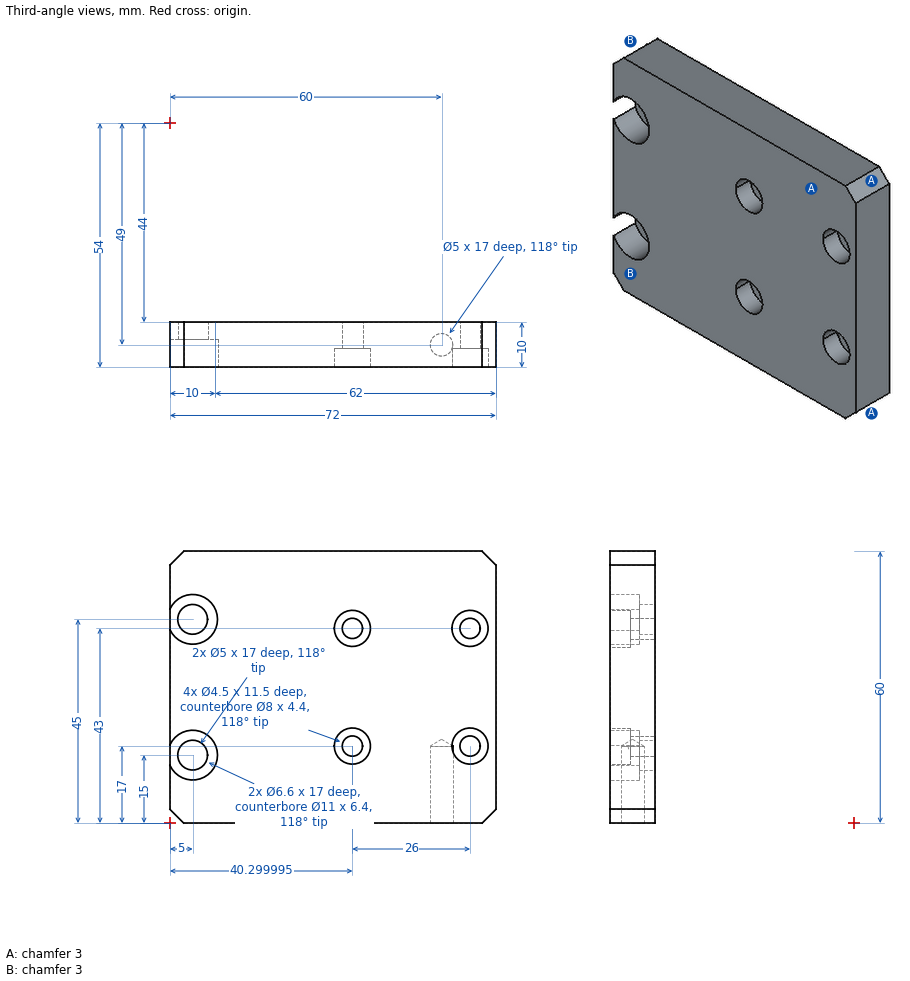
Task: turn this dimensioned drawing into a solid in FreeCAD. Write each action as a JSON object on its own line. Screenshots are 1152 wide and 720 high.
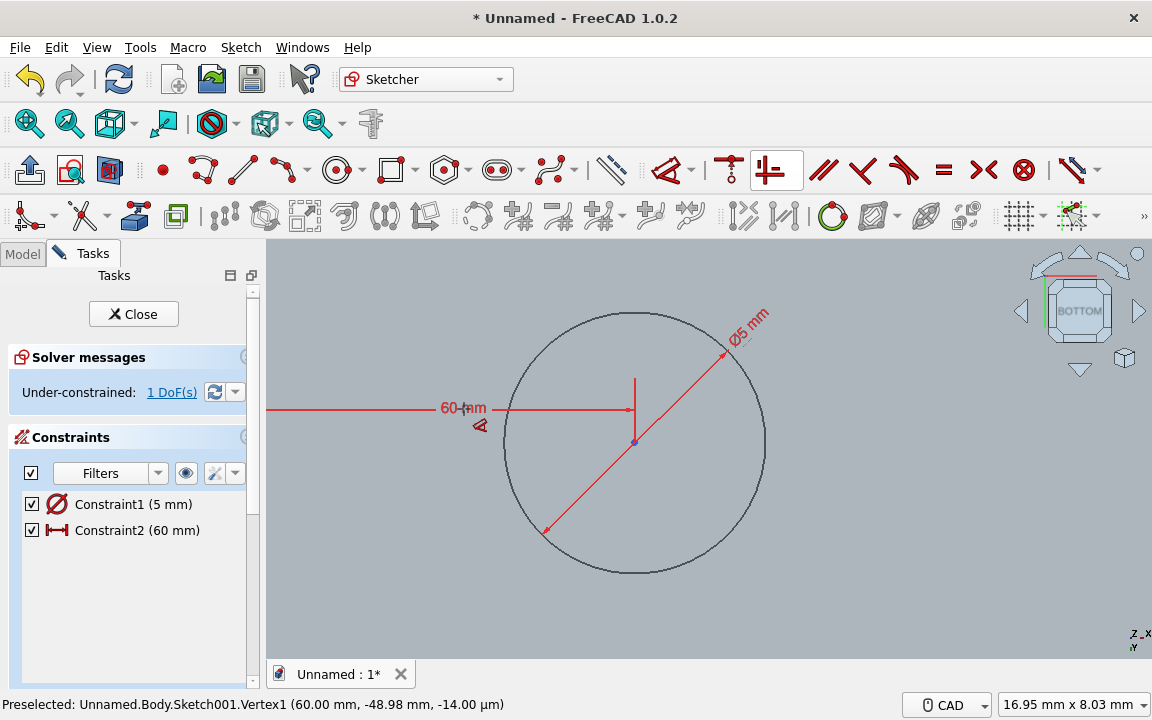
{"action": "left_click", "coordinate": [635, 443]}
{"action": "left_click", "coordinate": [669, 537]}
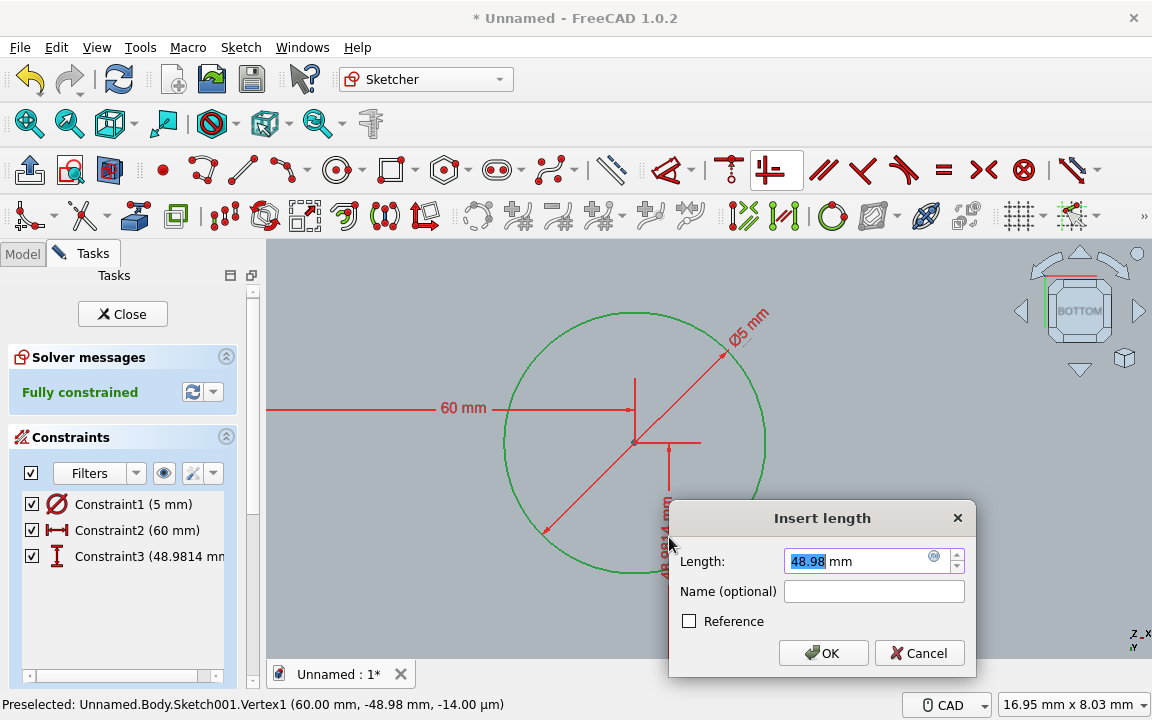
{"action": "type", "text": "49"}
{"action": "key", "text": "Return"}
{"action": "key", "text": "Escape"}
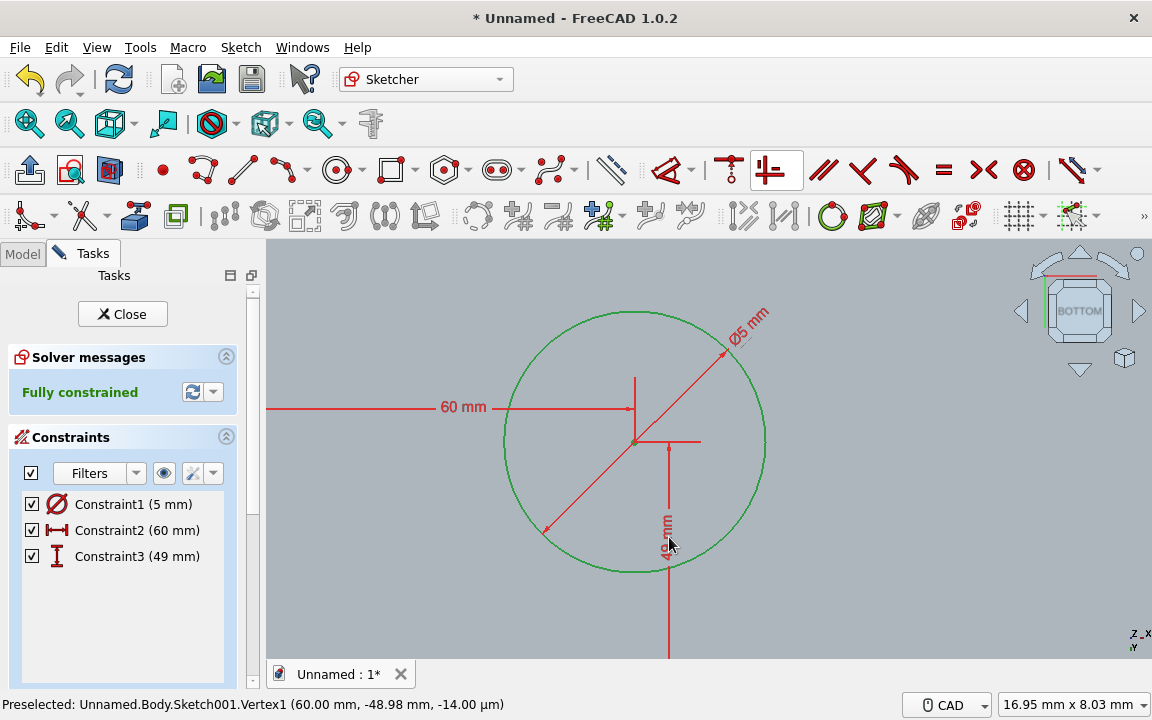
{"action": "left_click", "coordinate": [123, 314]}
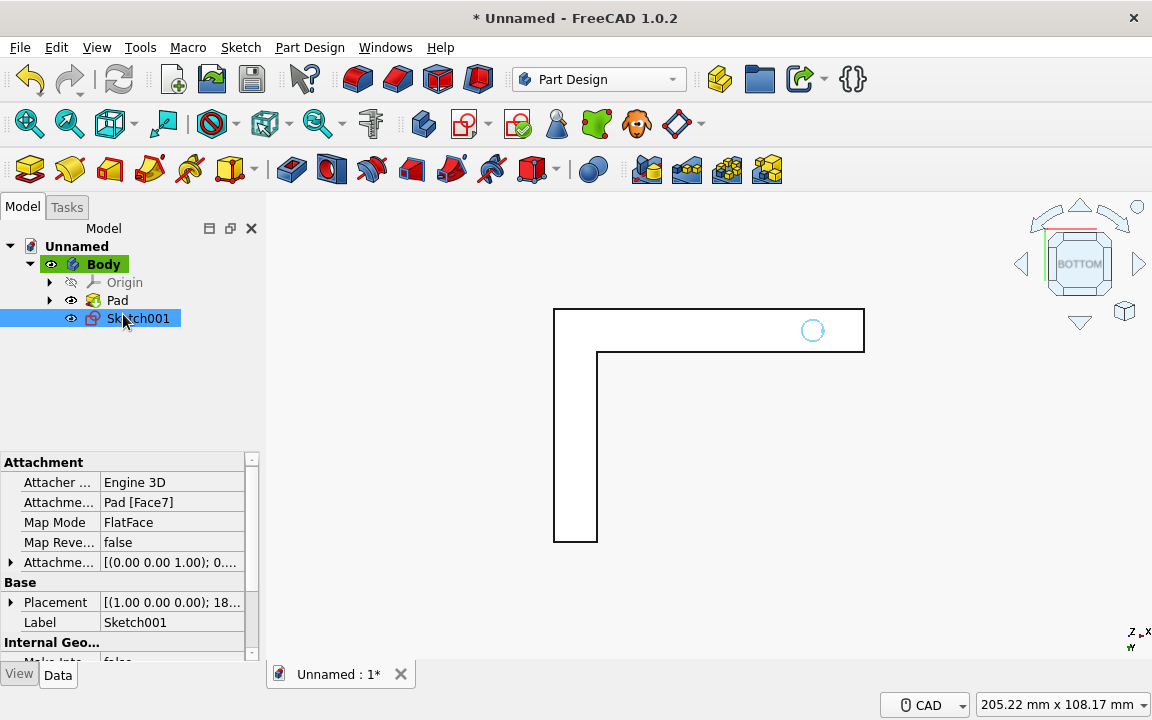
{"action": "left_click", "coordinate": [332, 170]}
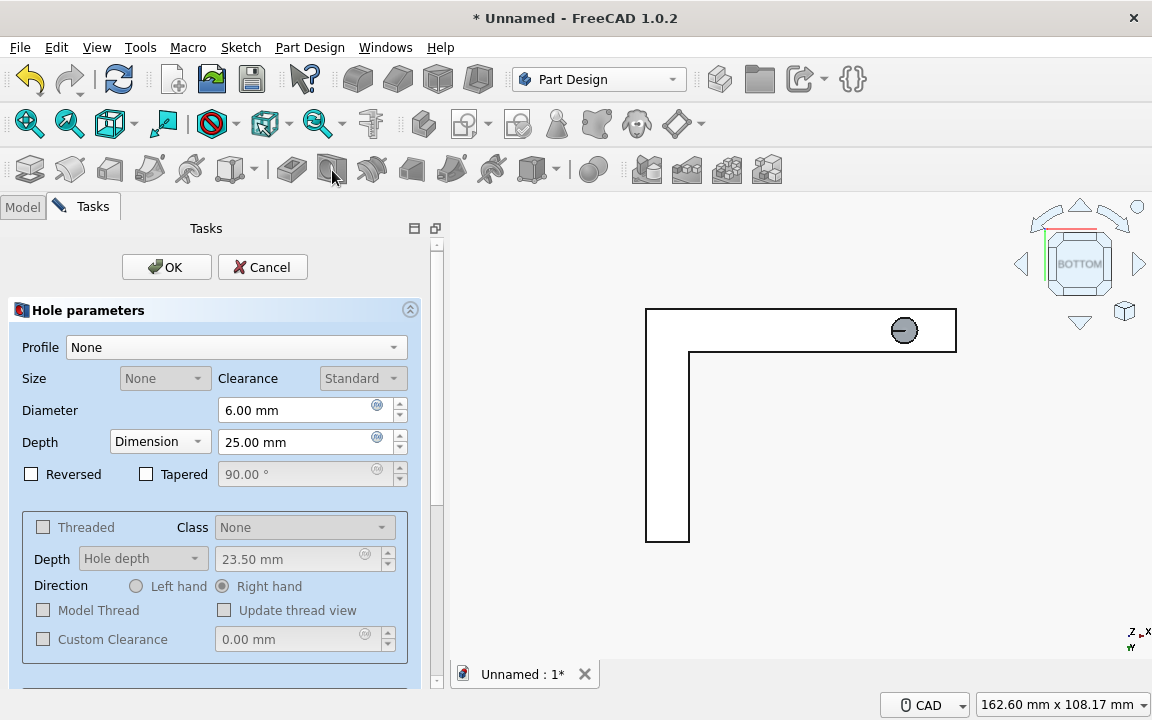
{"action": "triple_click", "coordinate": [305, 410]}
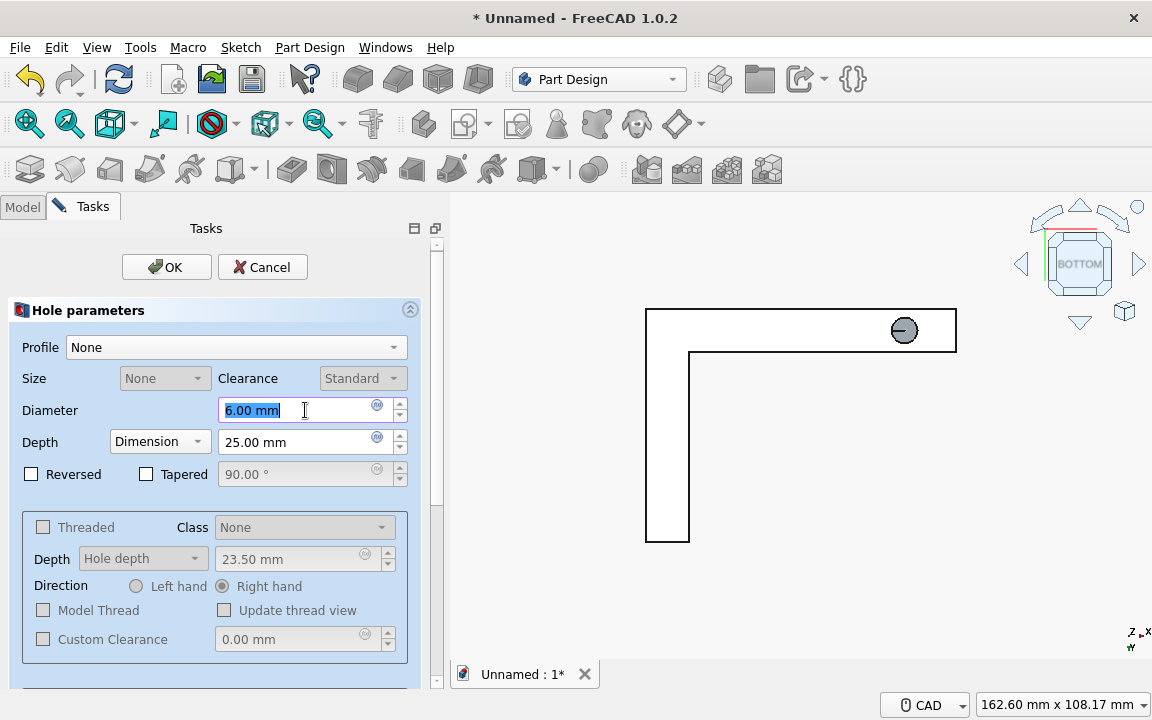
{"action": "type", "text": "5"}
{"action": "key", "text": "Tab"}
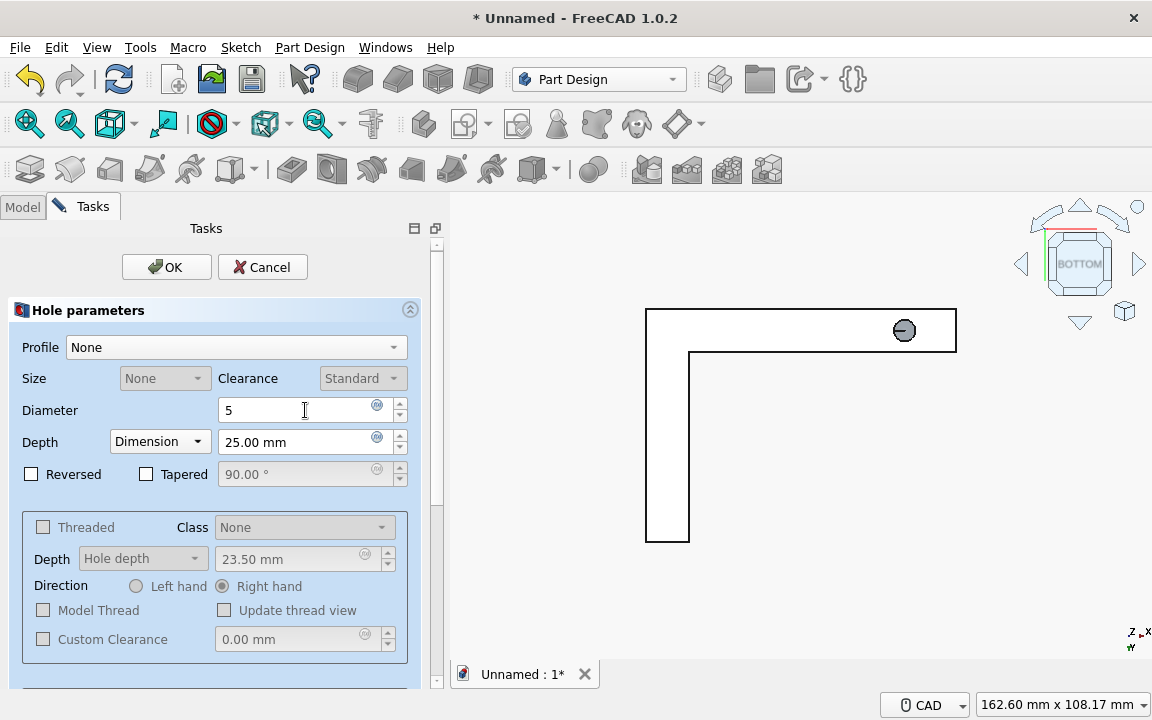
{"action": "triple_click", "coordinate": [305, 442]}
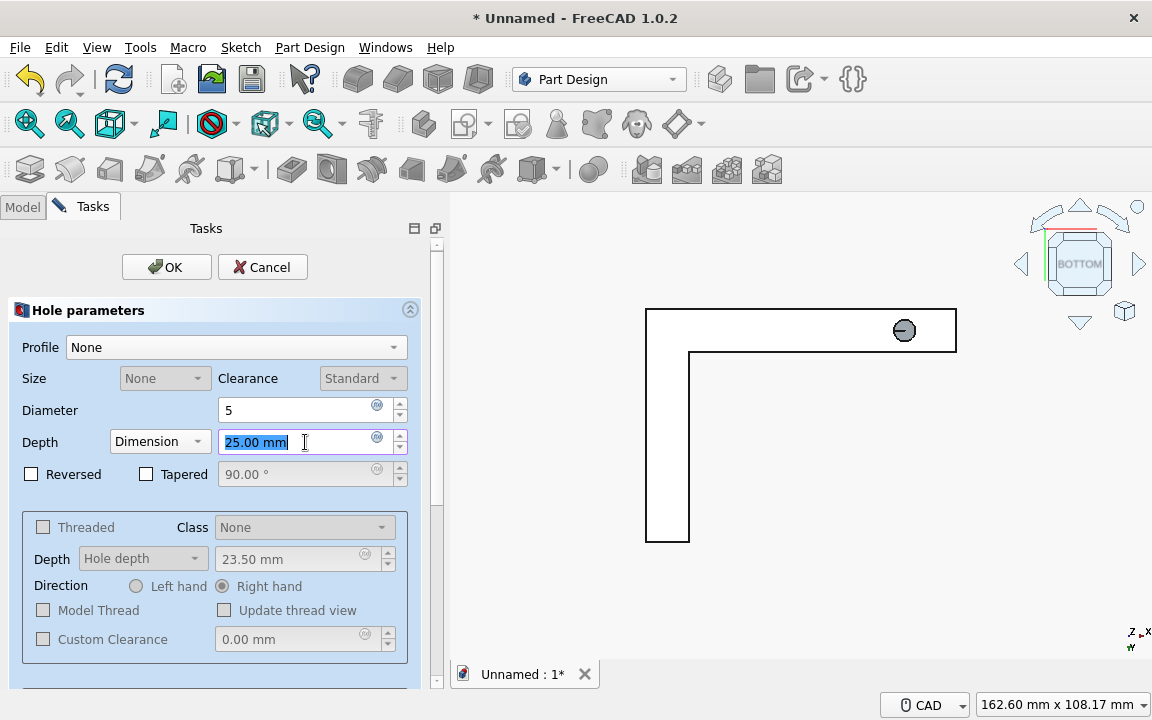
{"action": "type", "text": "17"}
{"action": "key", "text": "Tab"}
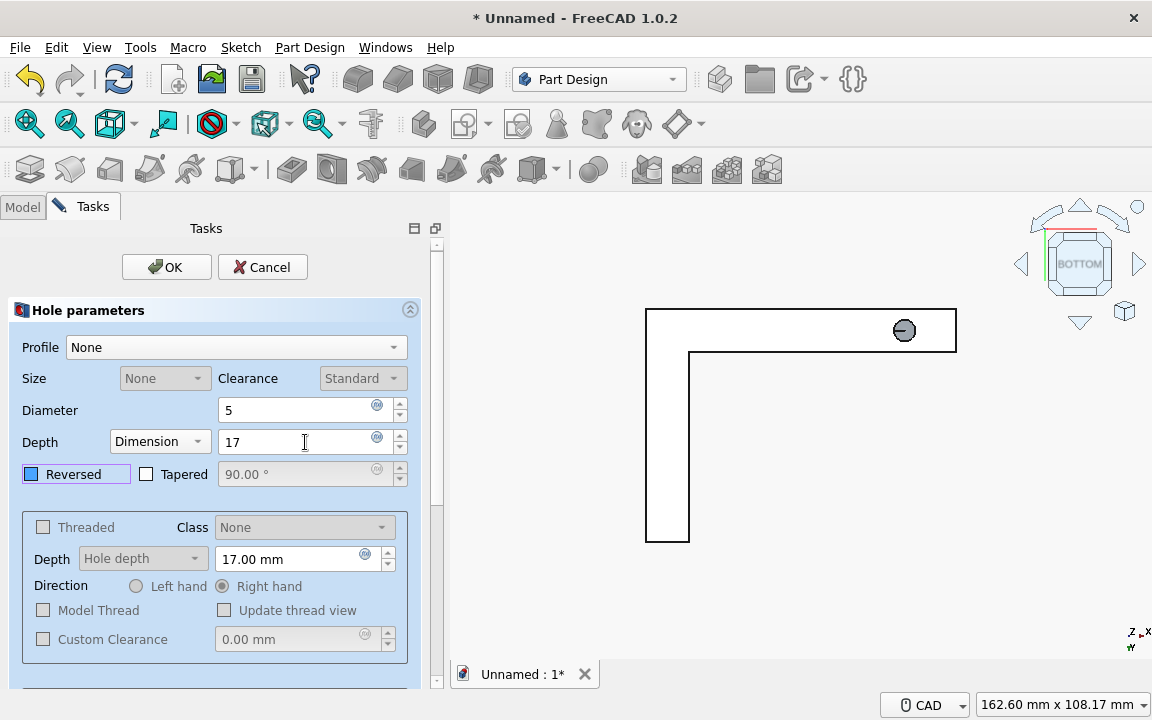
{"action": "left_click", "coordinate": [167, 267]}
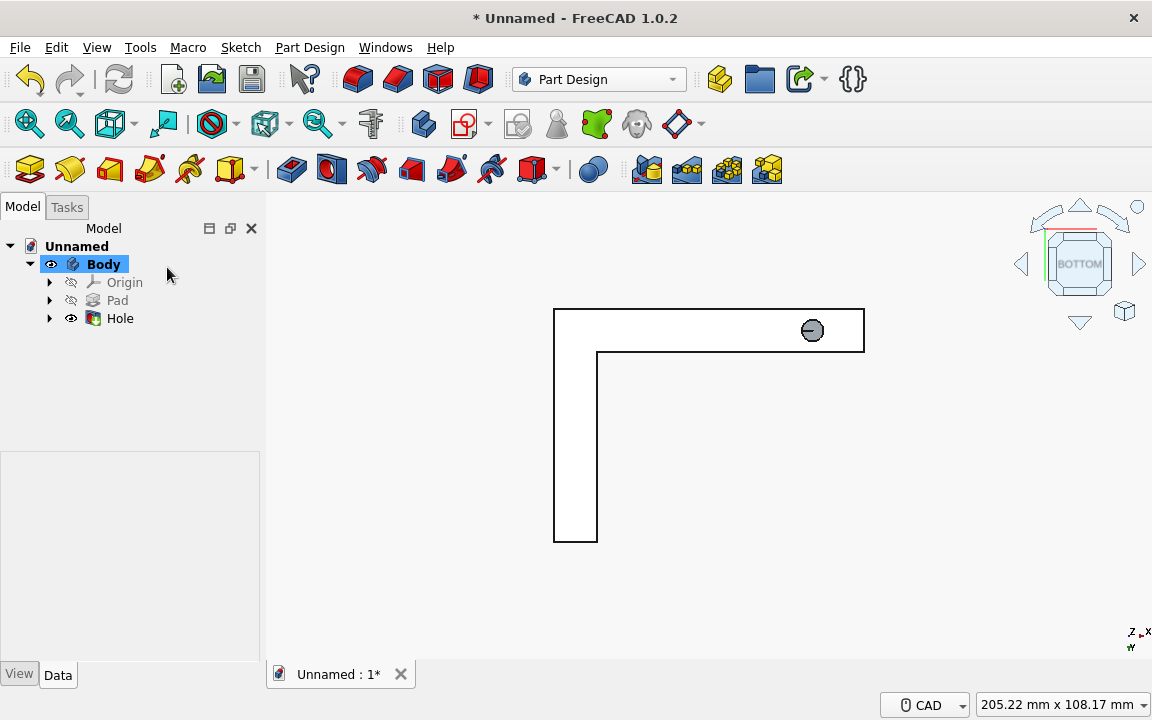
{"action": "key", "text": "0"}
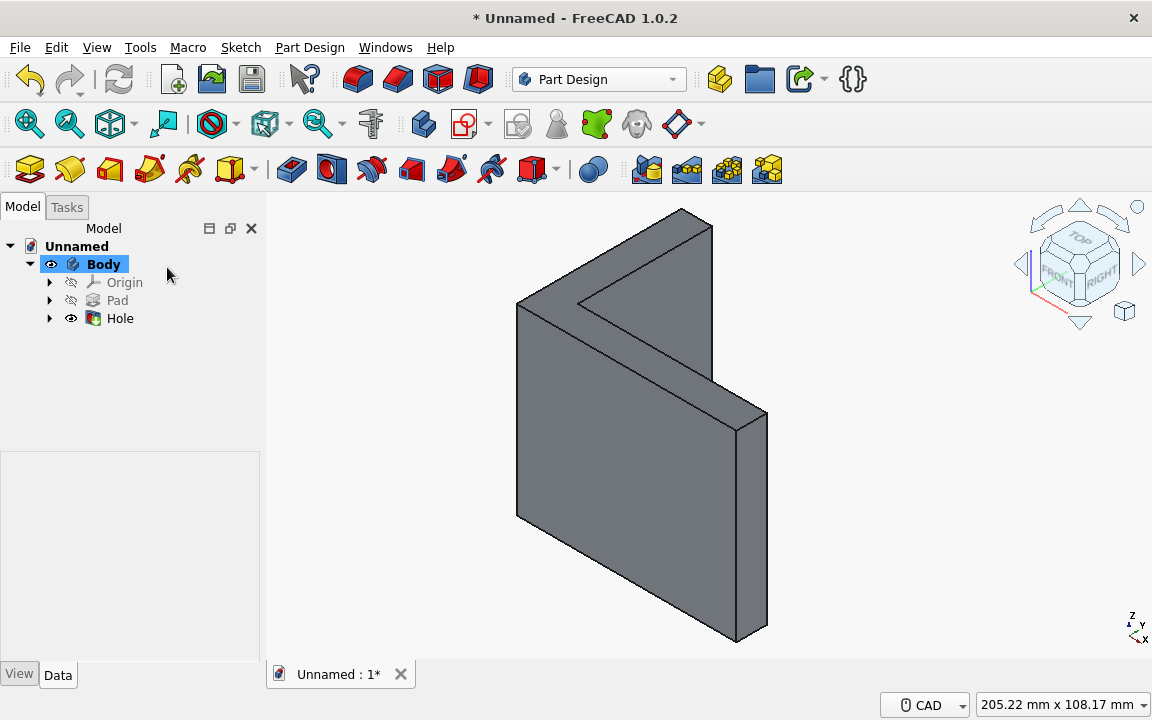
{"action": "left_click", "coordinate": [627, 472]}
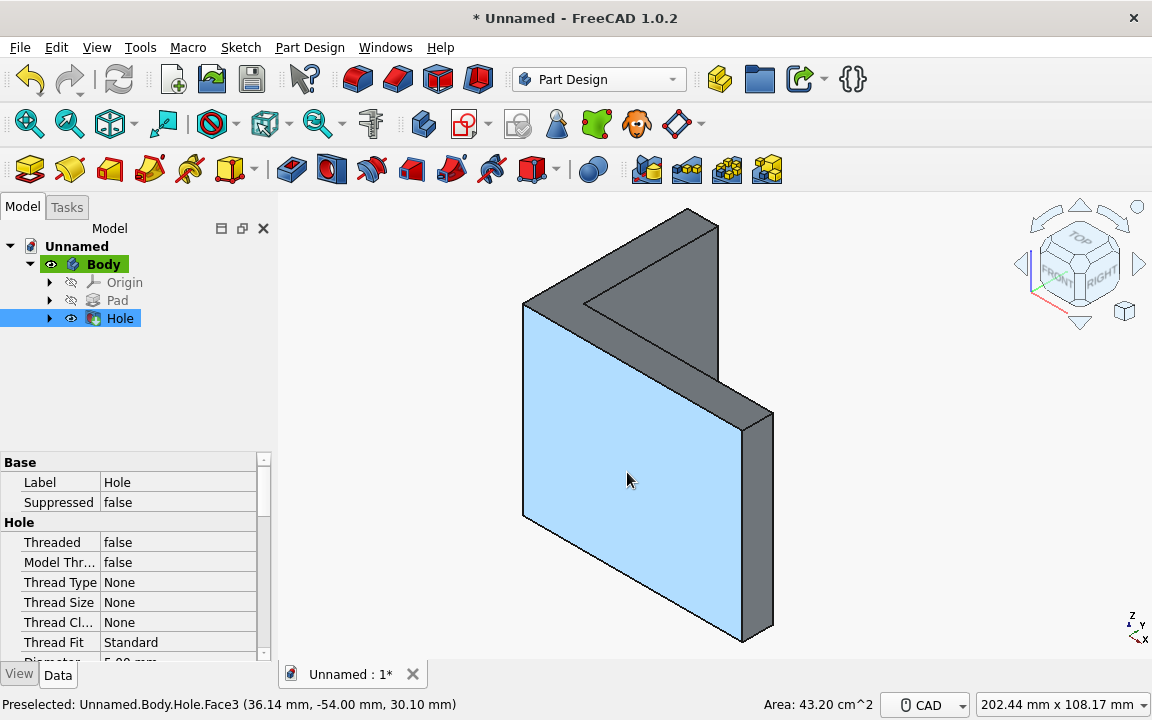
{"action": "left_click", "coordinate": [464, 124]}